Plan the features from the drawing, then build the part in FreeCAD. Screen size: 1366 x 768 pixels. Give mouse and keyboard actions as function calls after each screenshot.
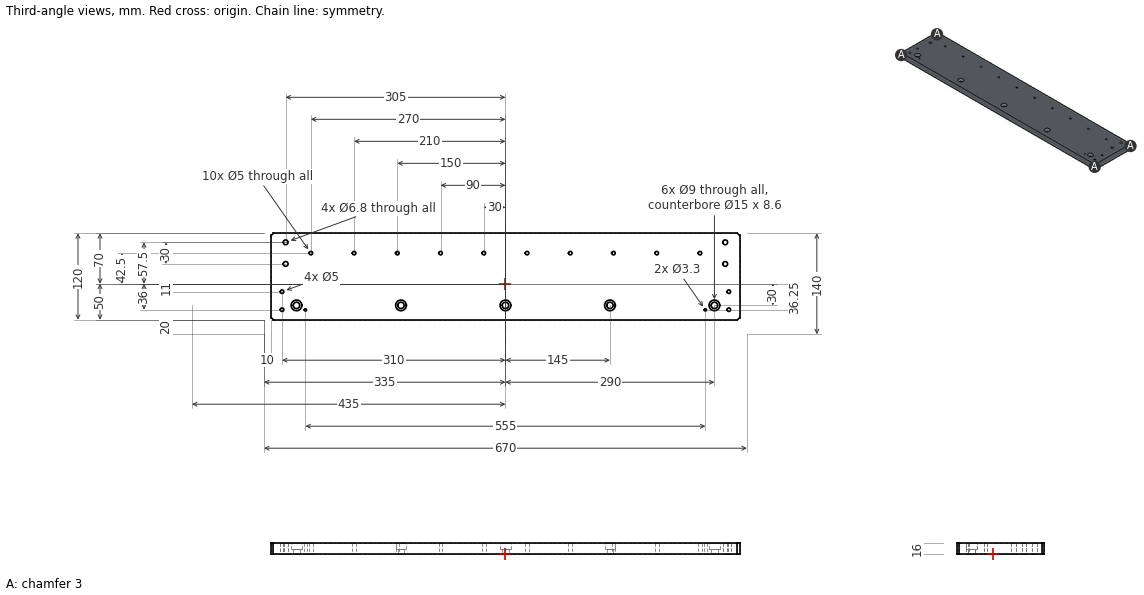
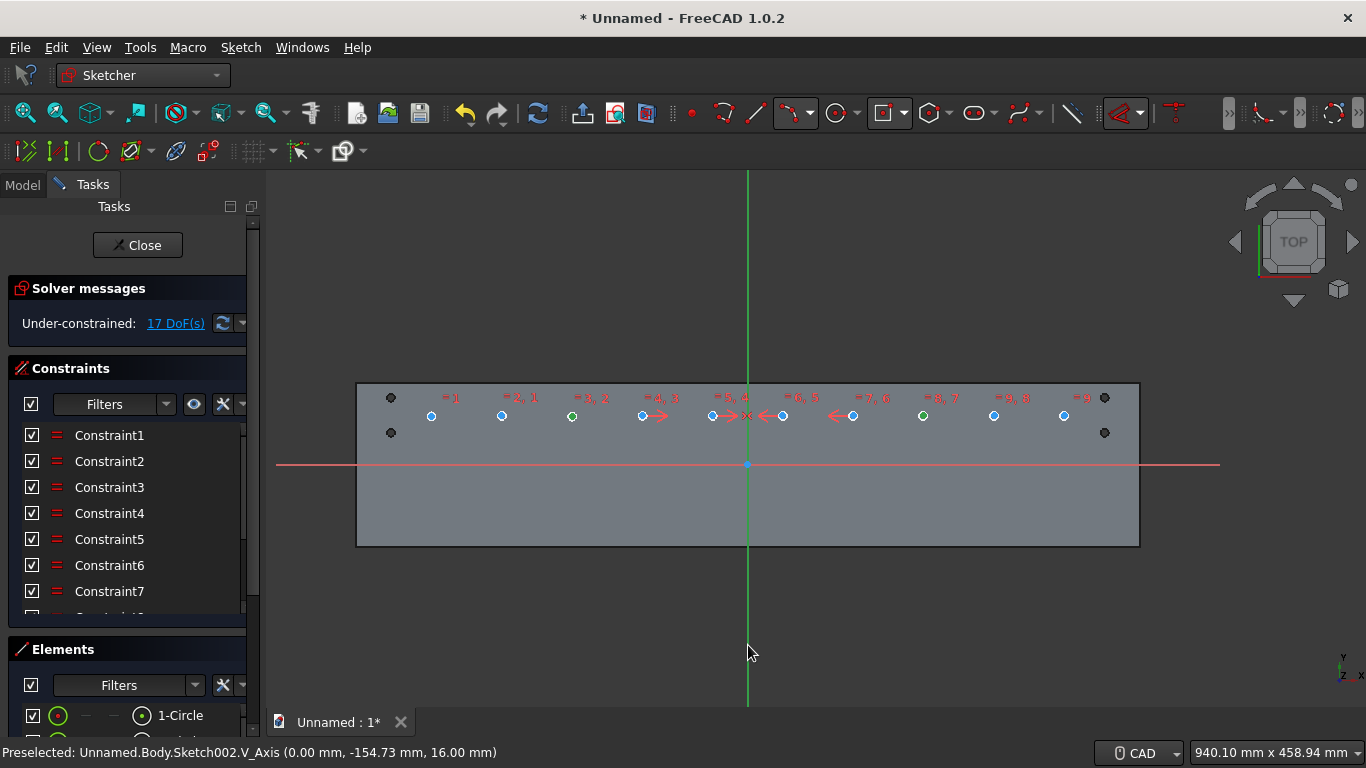
key(s)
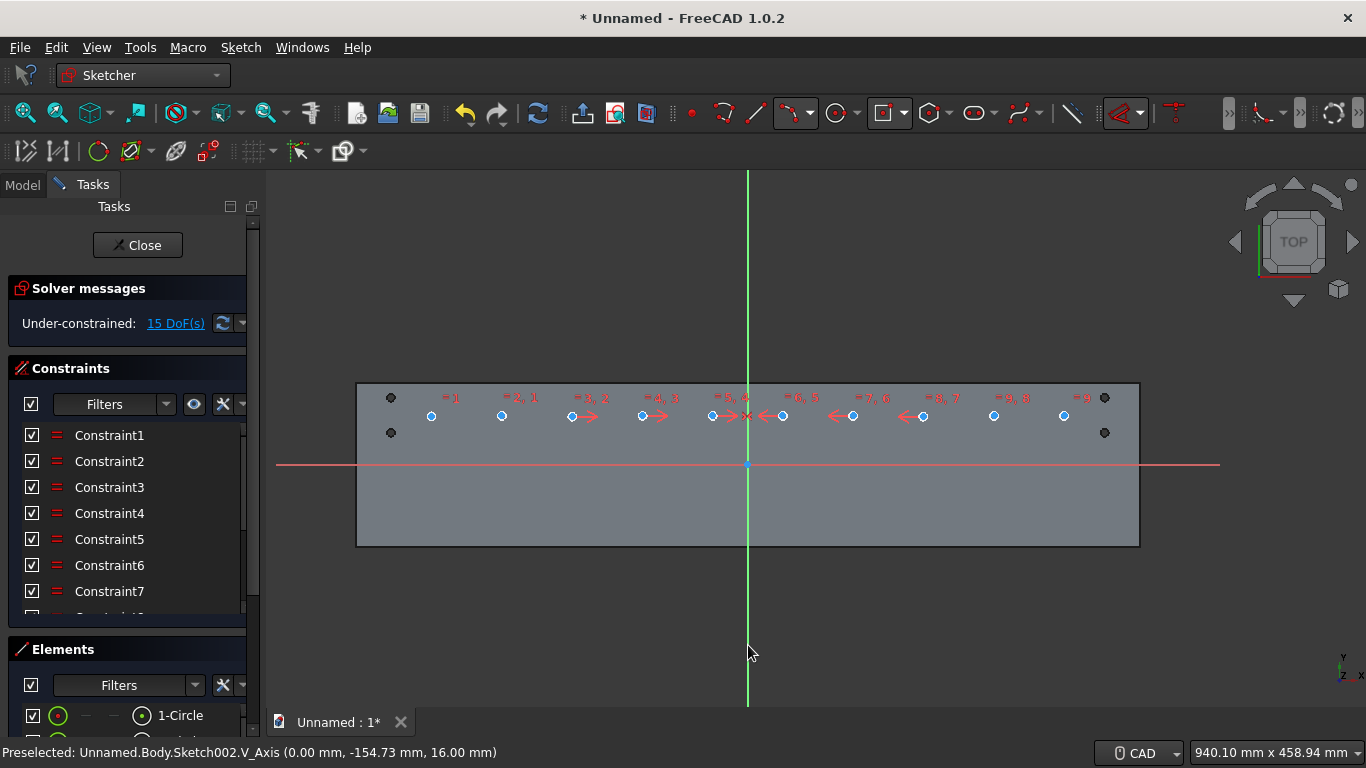
click(502, 416)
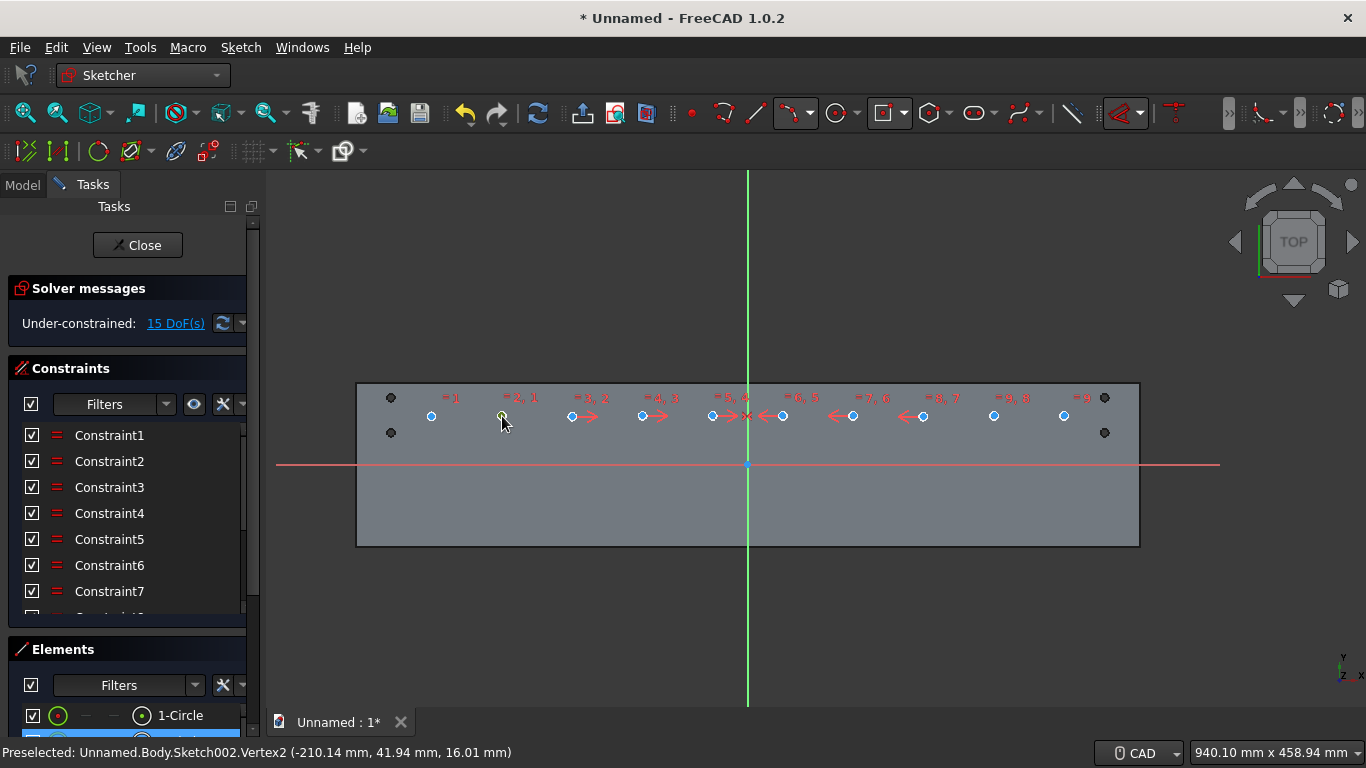
click(994, 416)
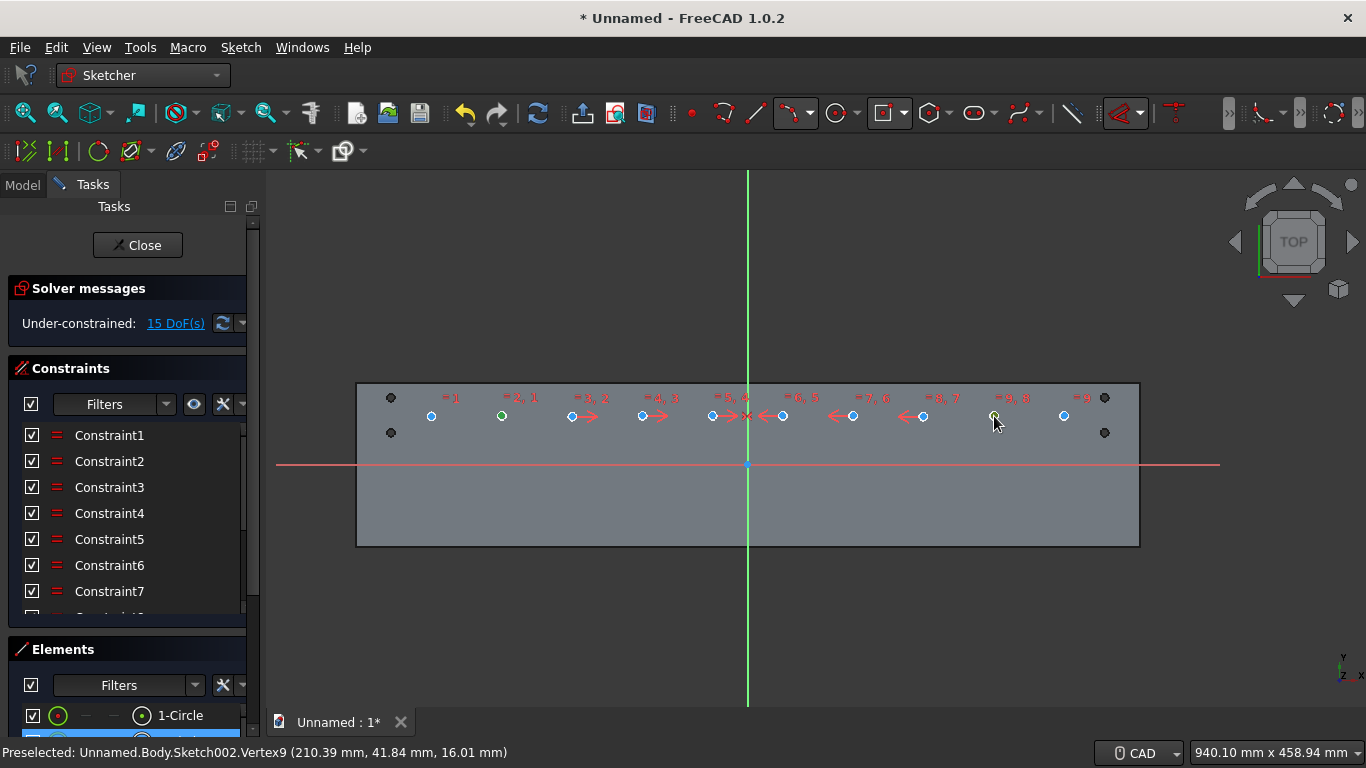
click(748, 645)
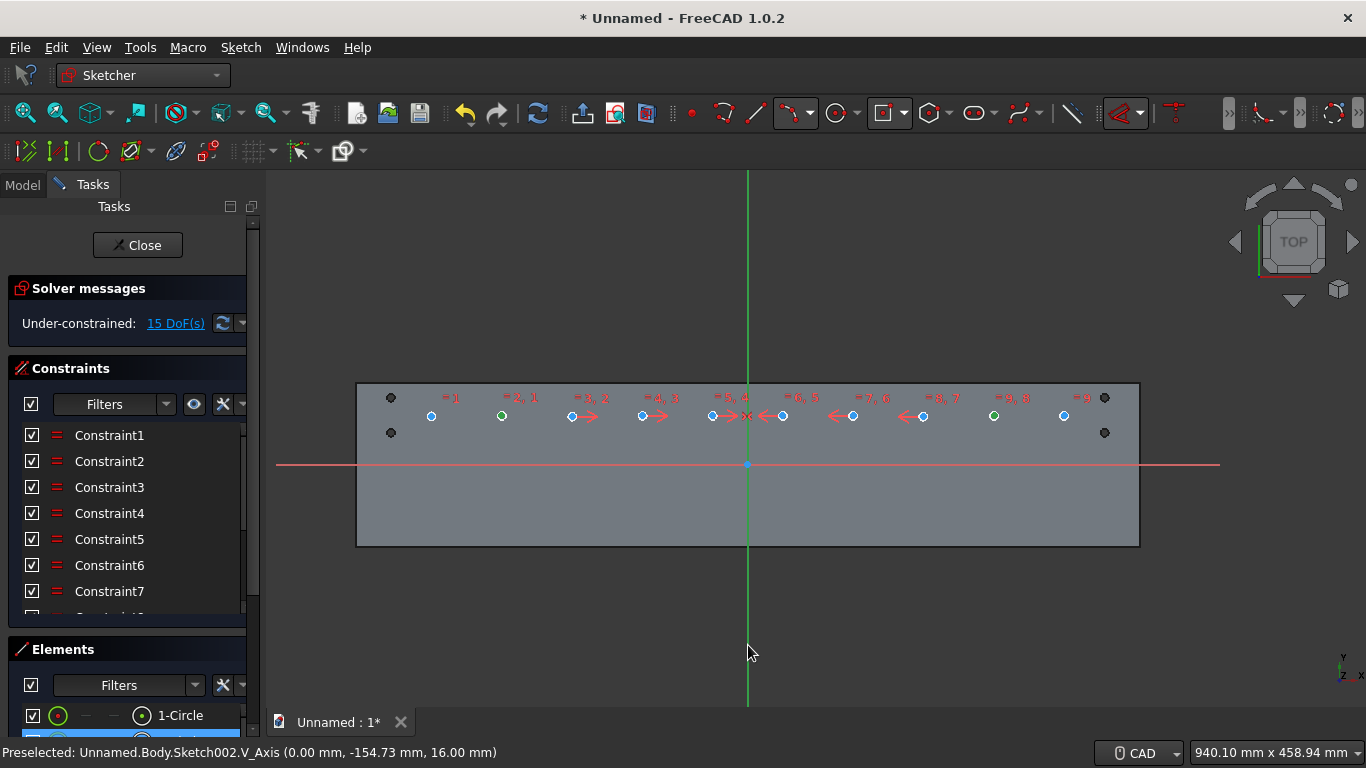
key(s)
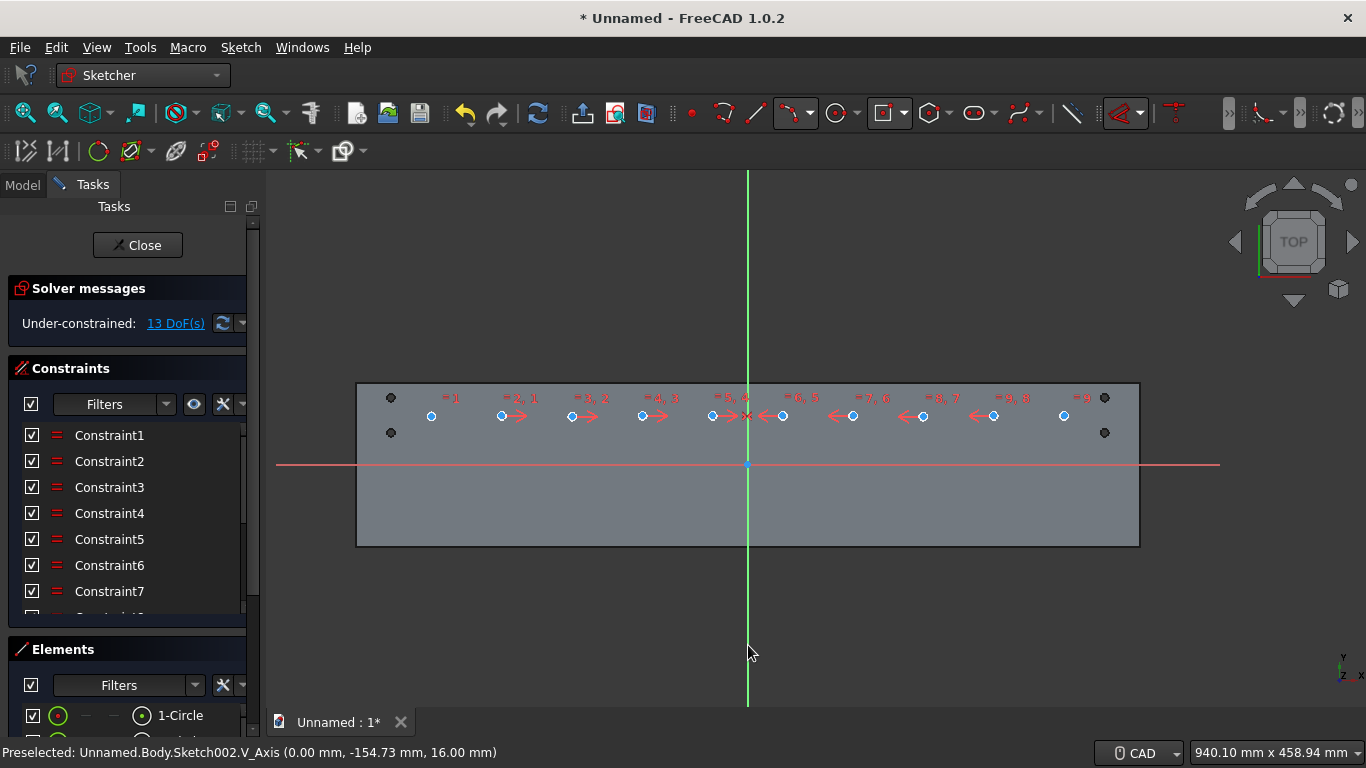
click(432, 416)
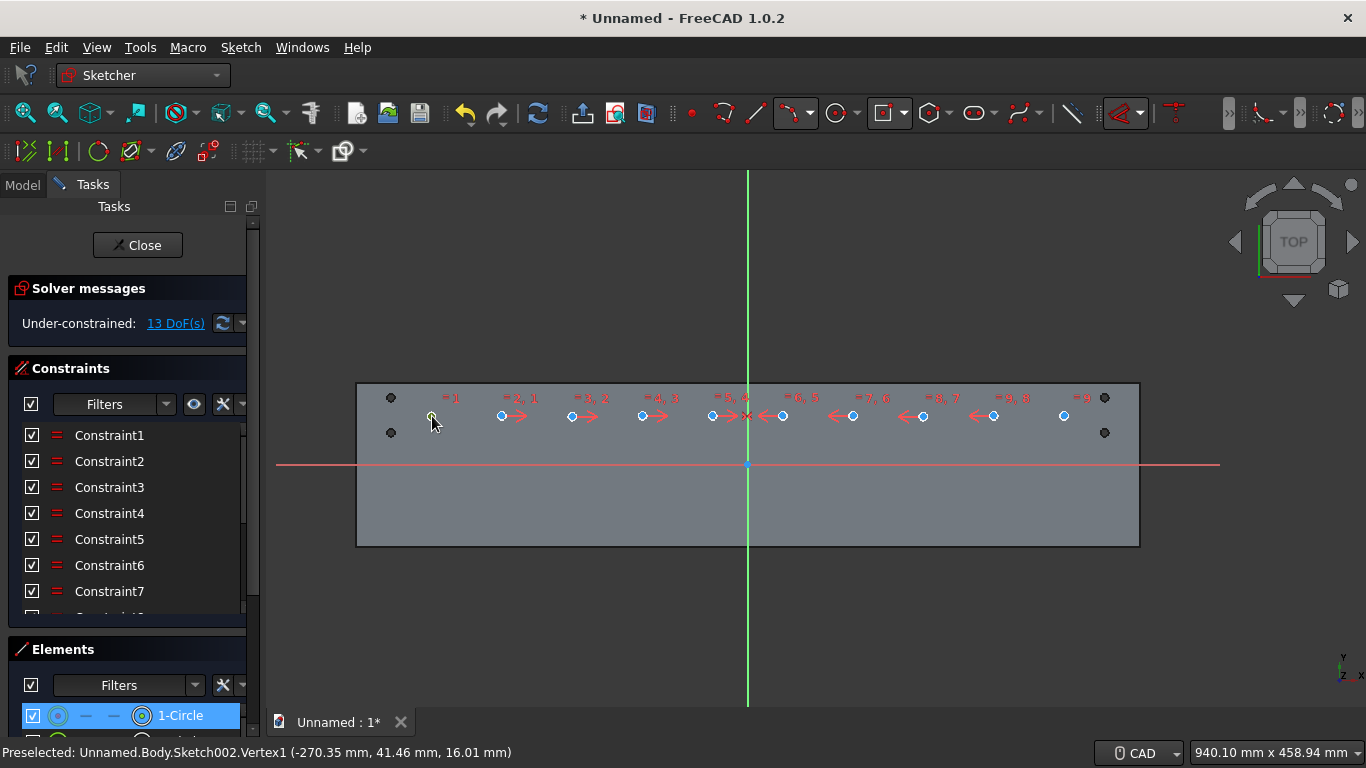
click(1064, 416)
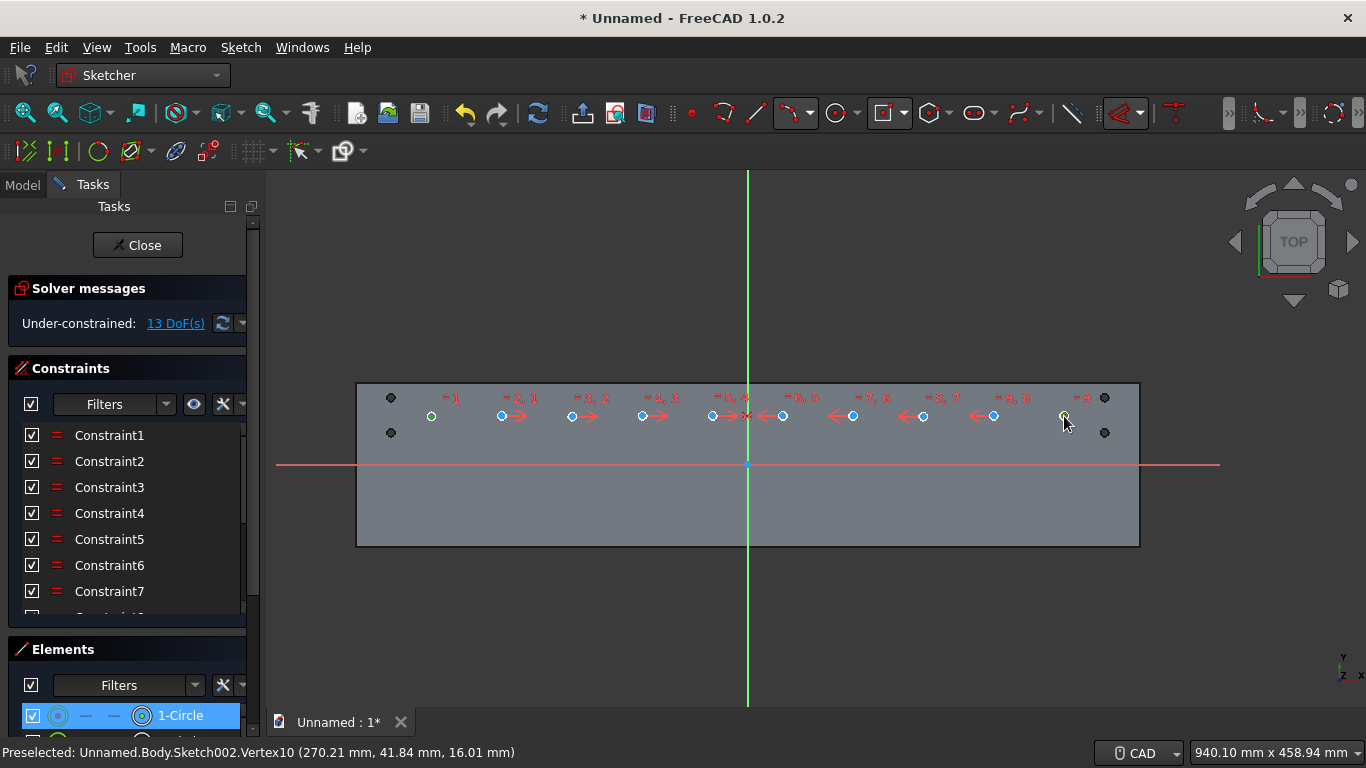
click(748, 645)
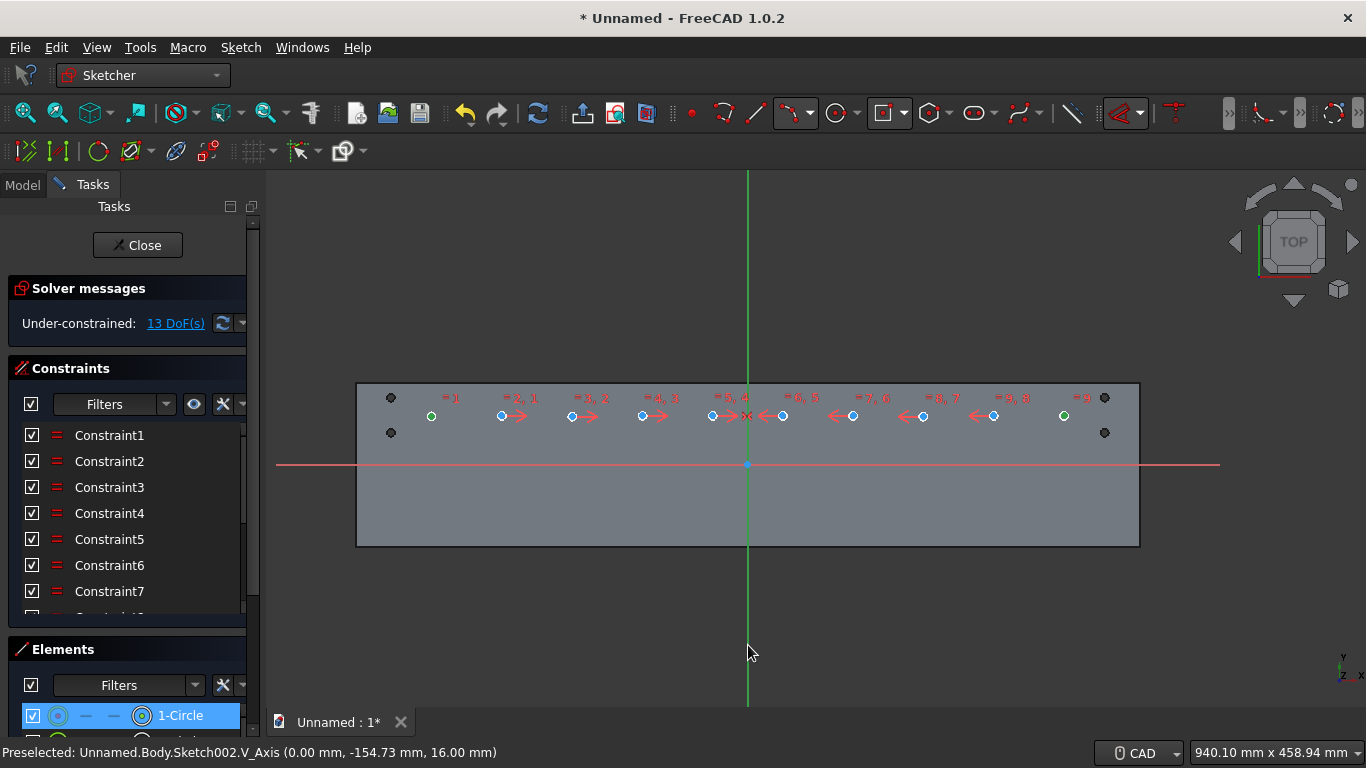
key(s)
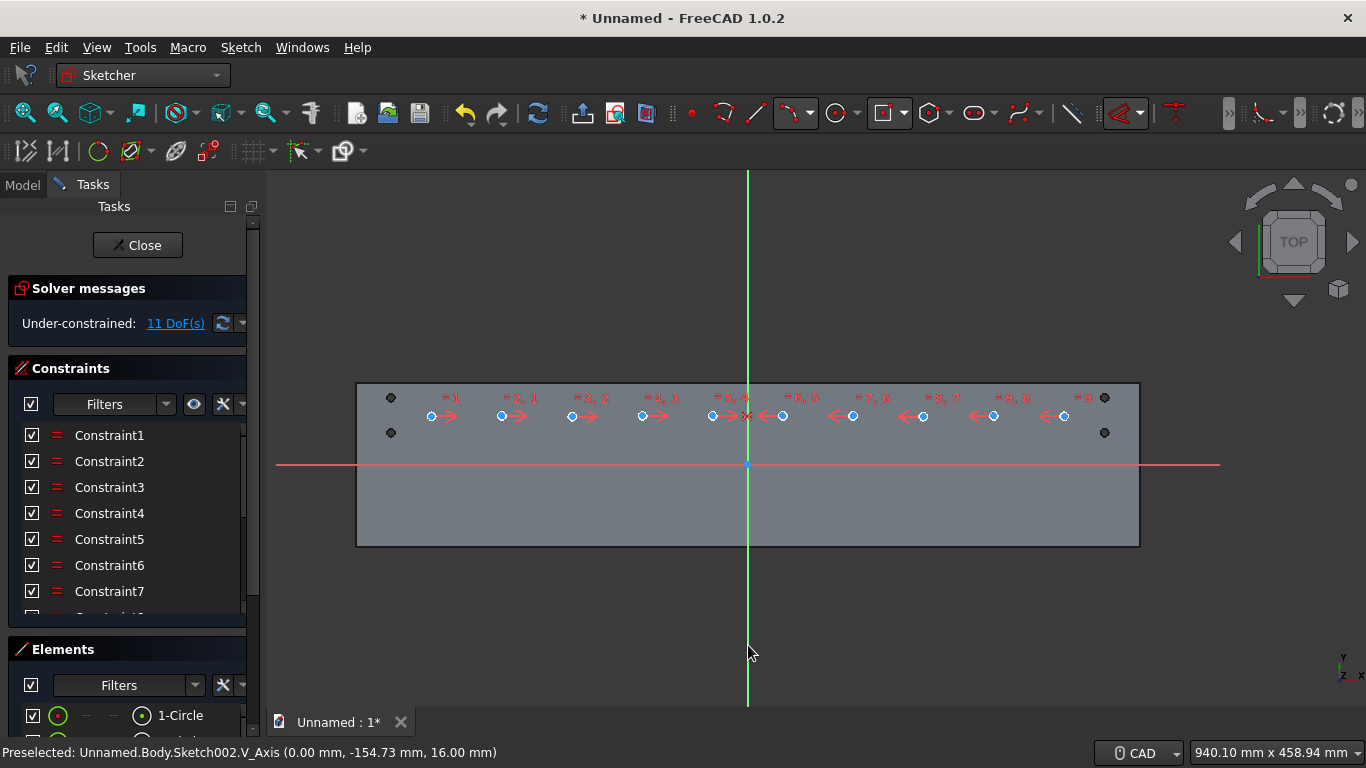
scroll(429, 414, up, 10)